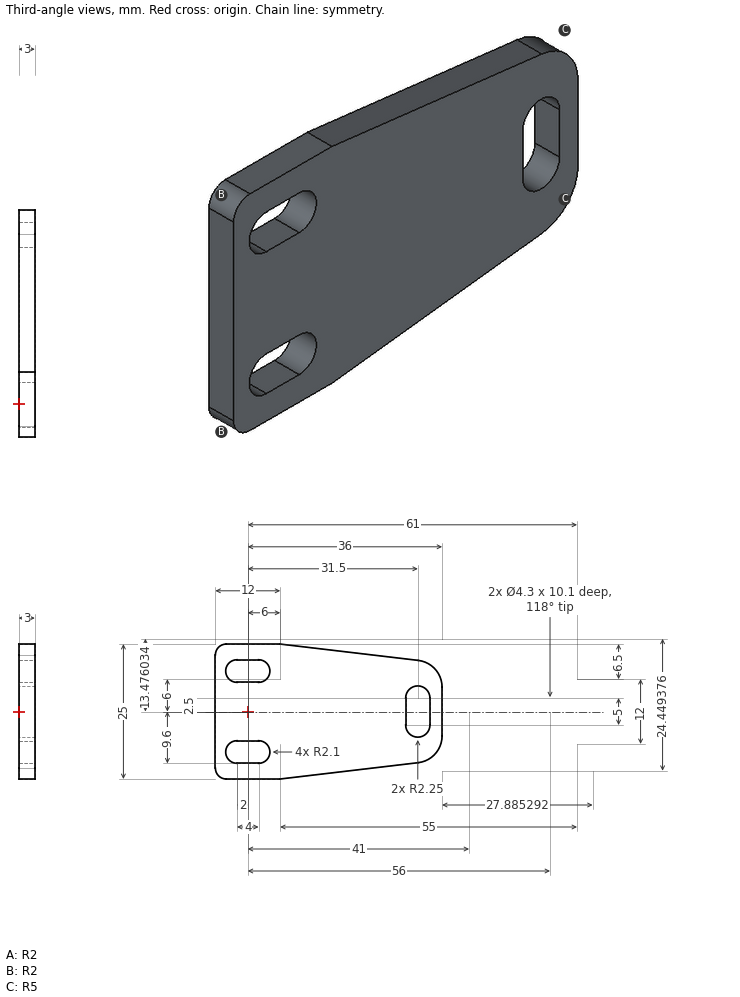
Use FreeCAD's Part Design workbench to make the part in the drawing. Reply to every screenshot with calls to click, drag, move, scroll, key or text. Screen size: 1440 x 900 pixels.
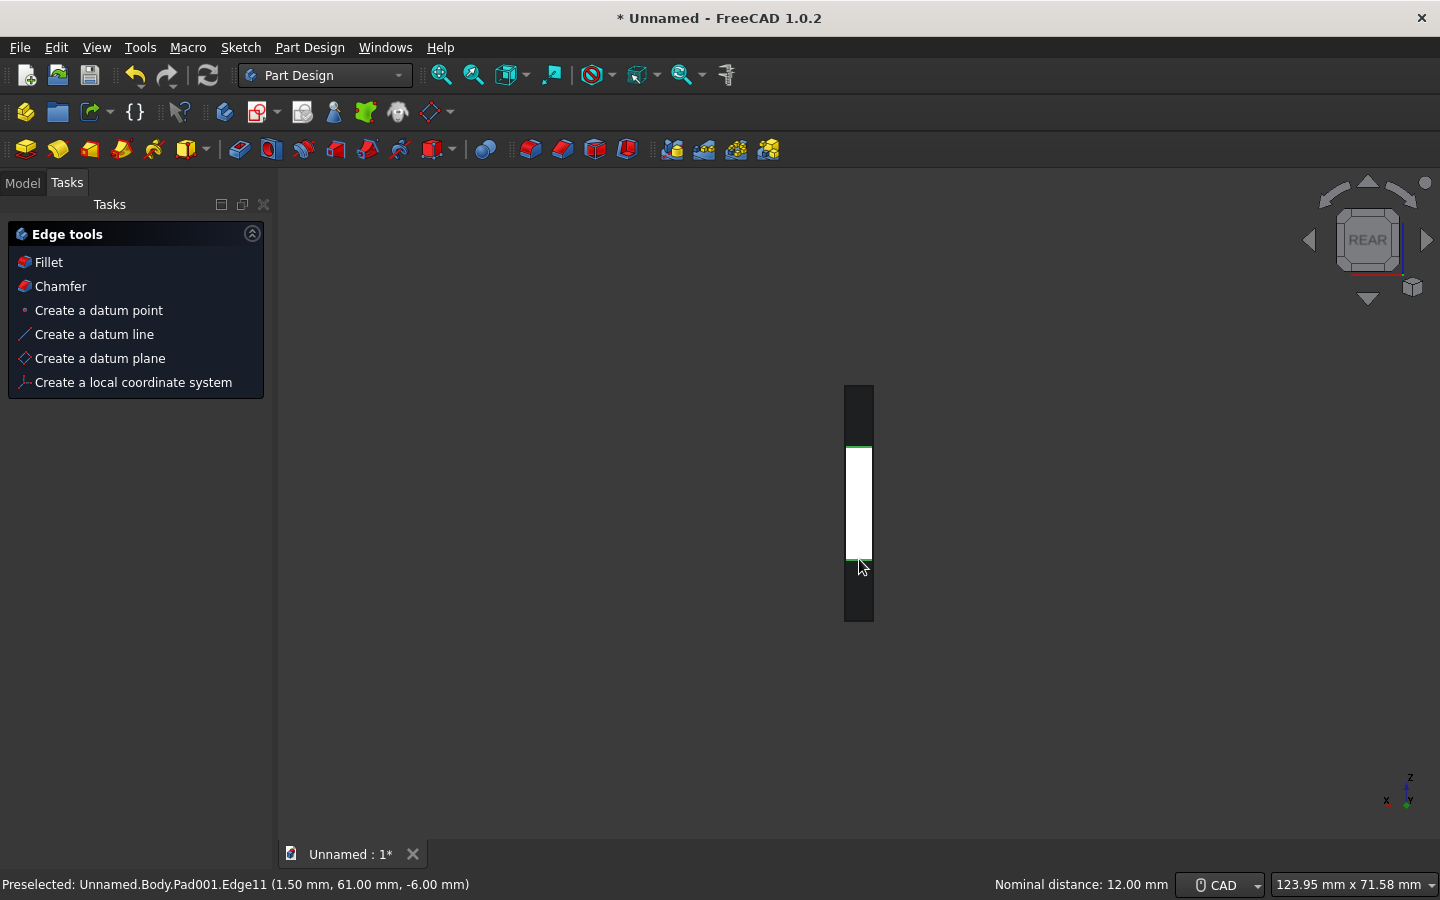
click(532, 150)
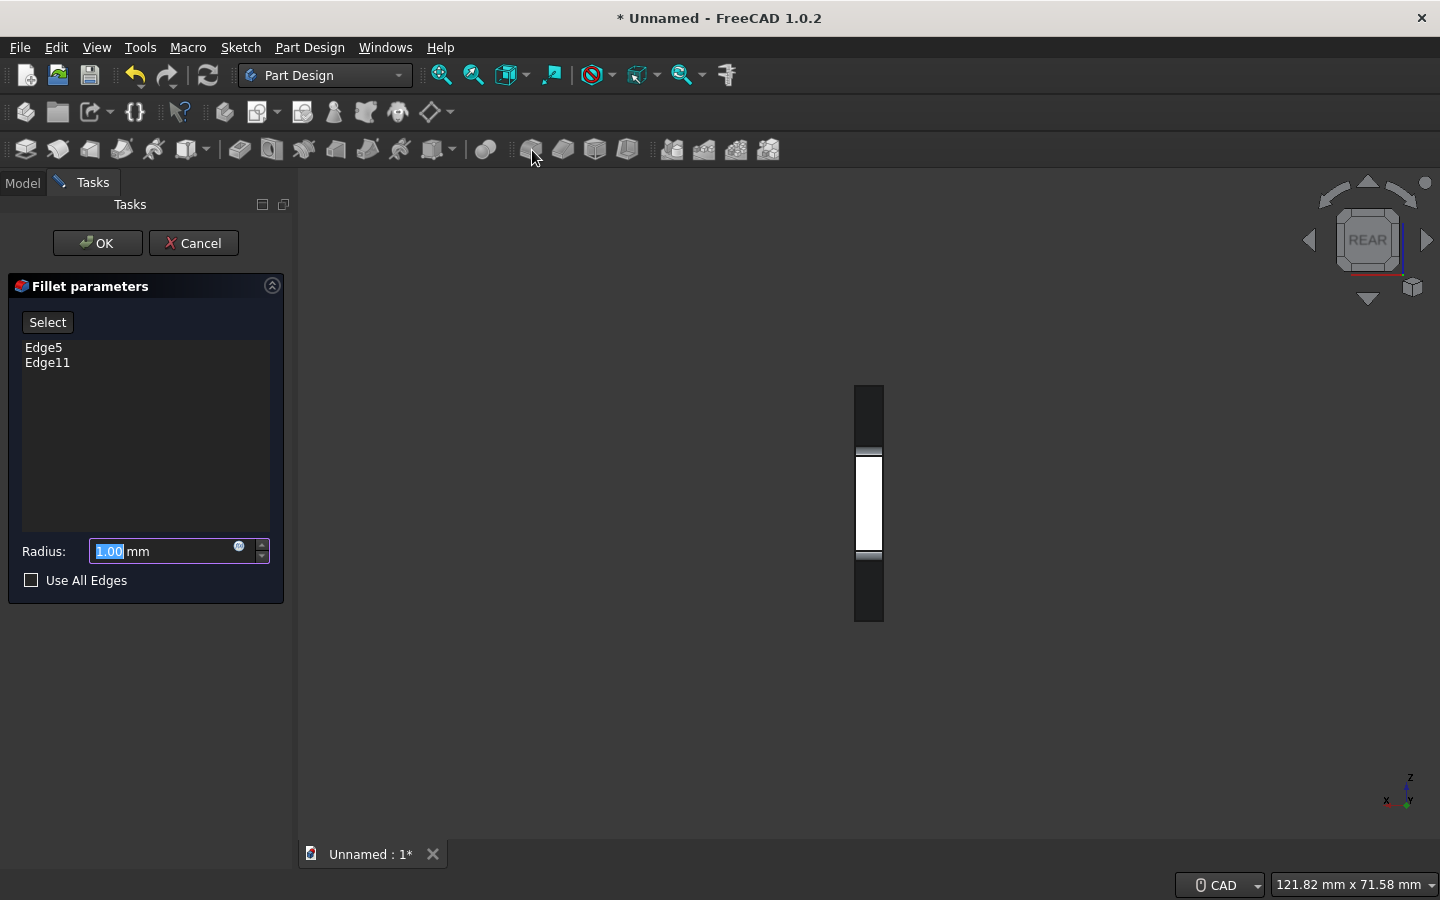
text(2)
key(Tab)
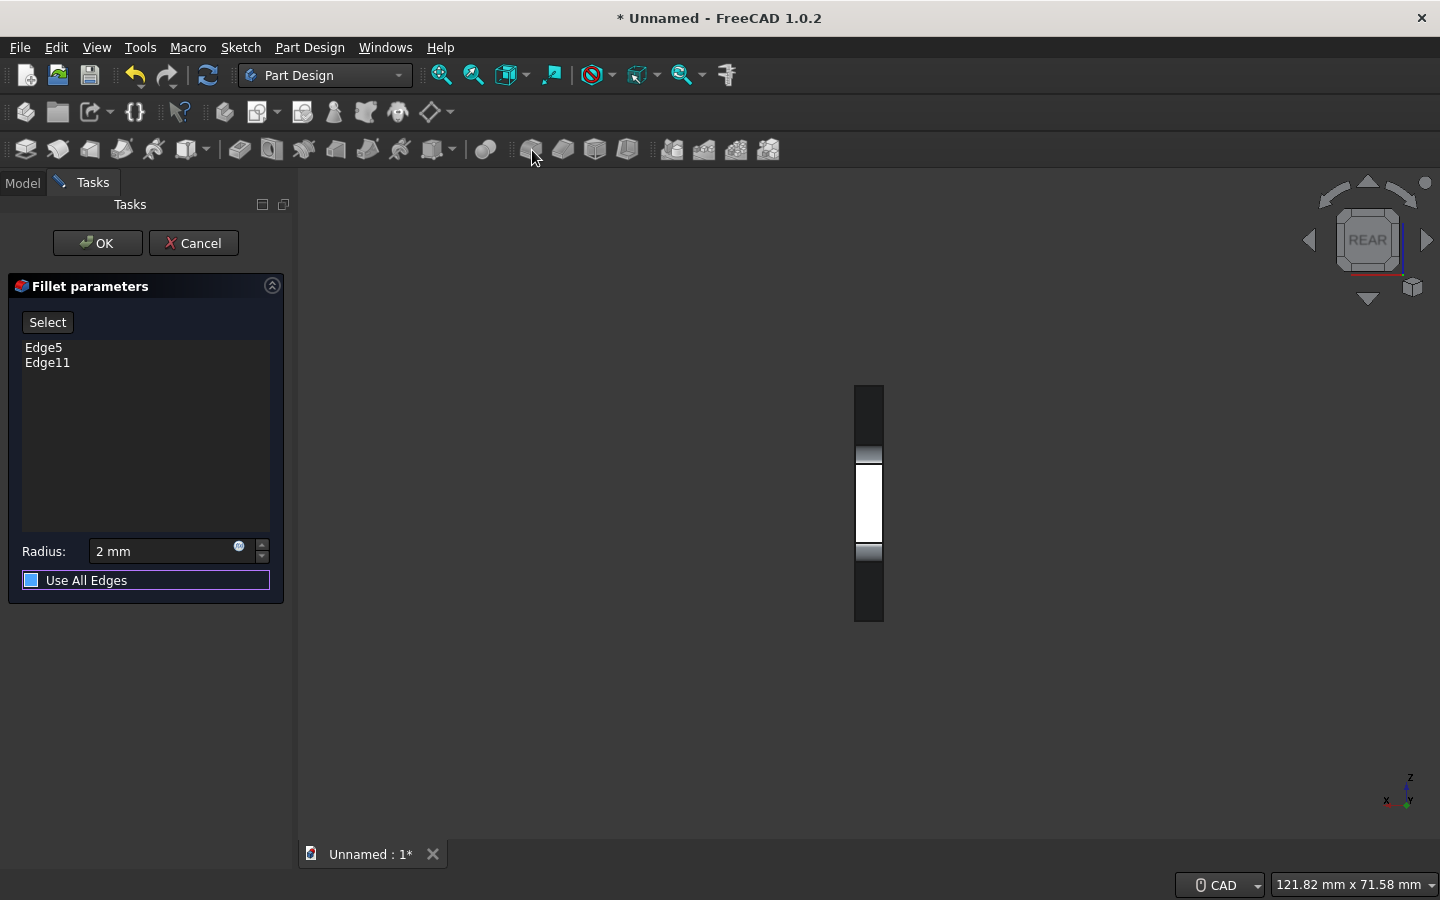
click(98, 243)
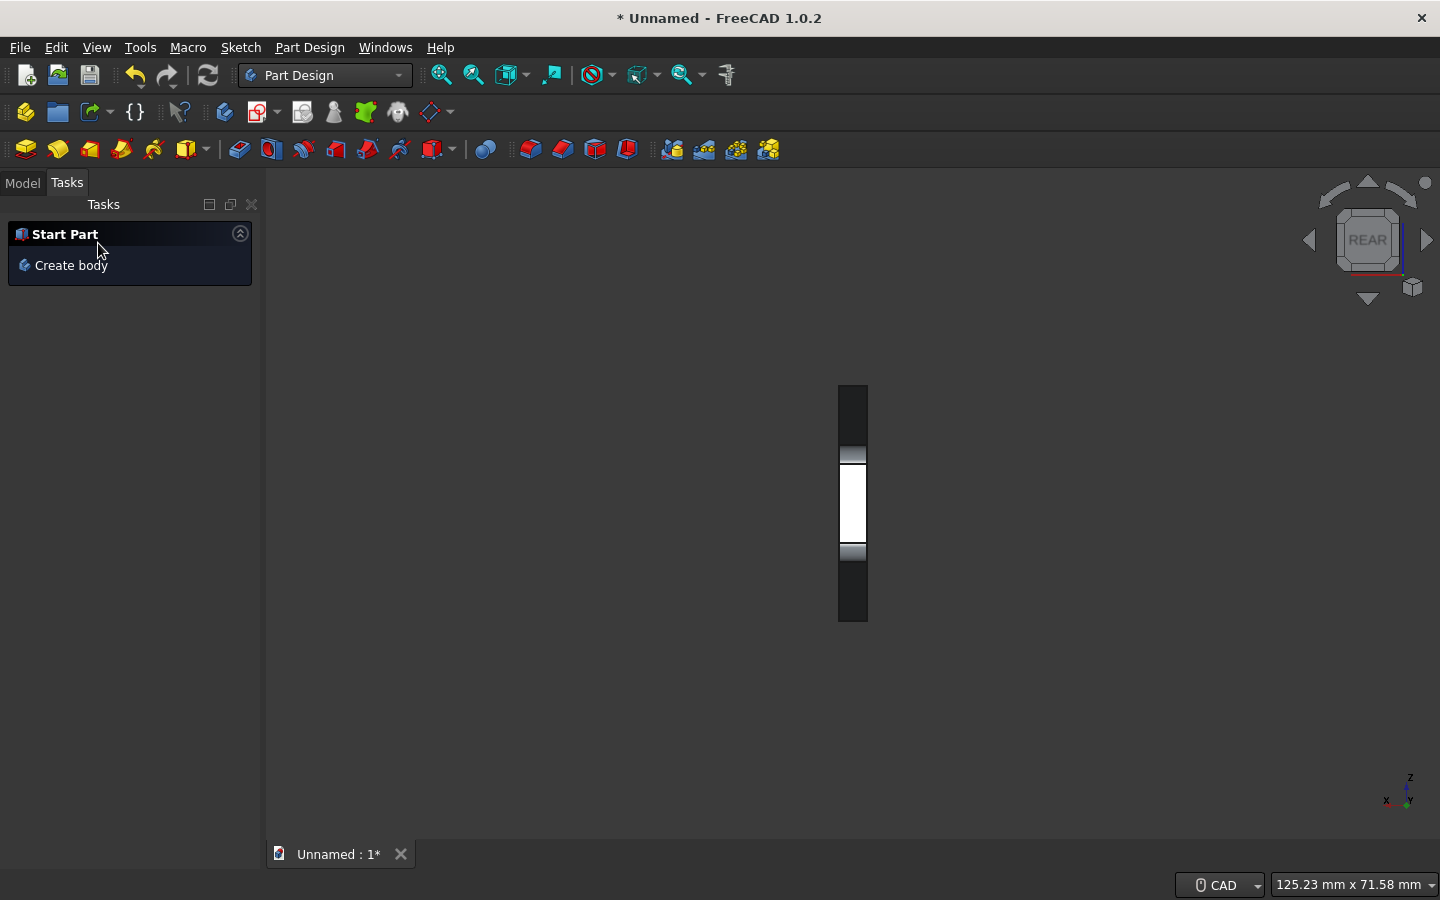
key(v)
key(f)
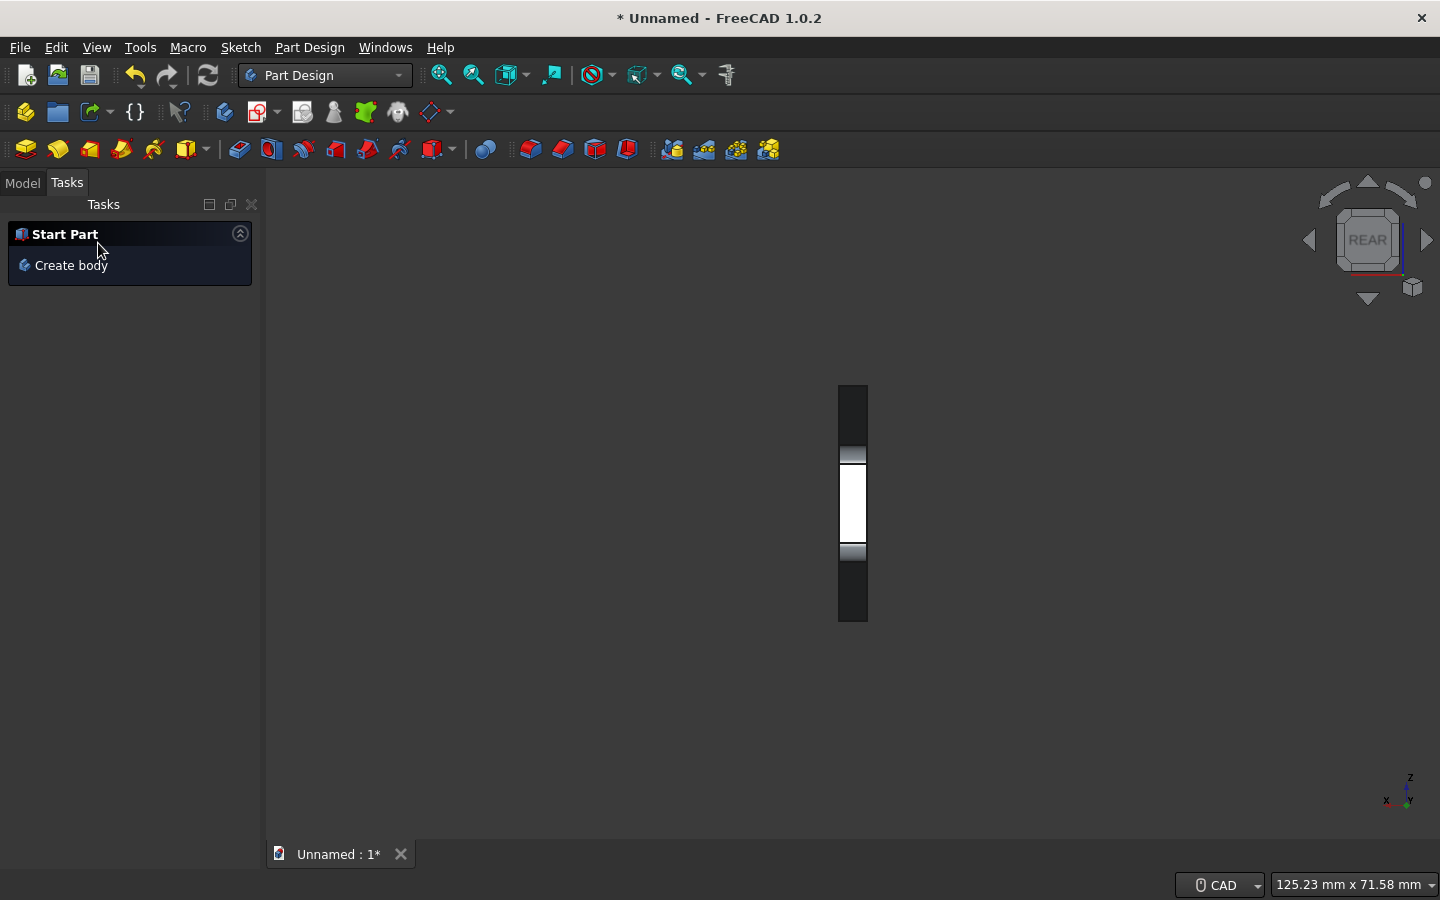
key(6)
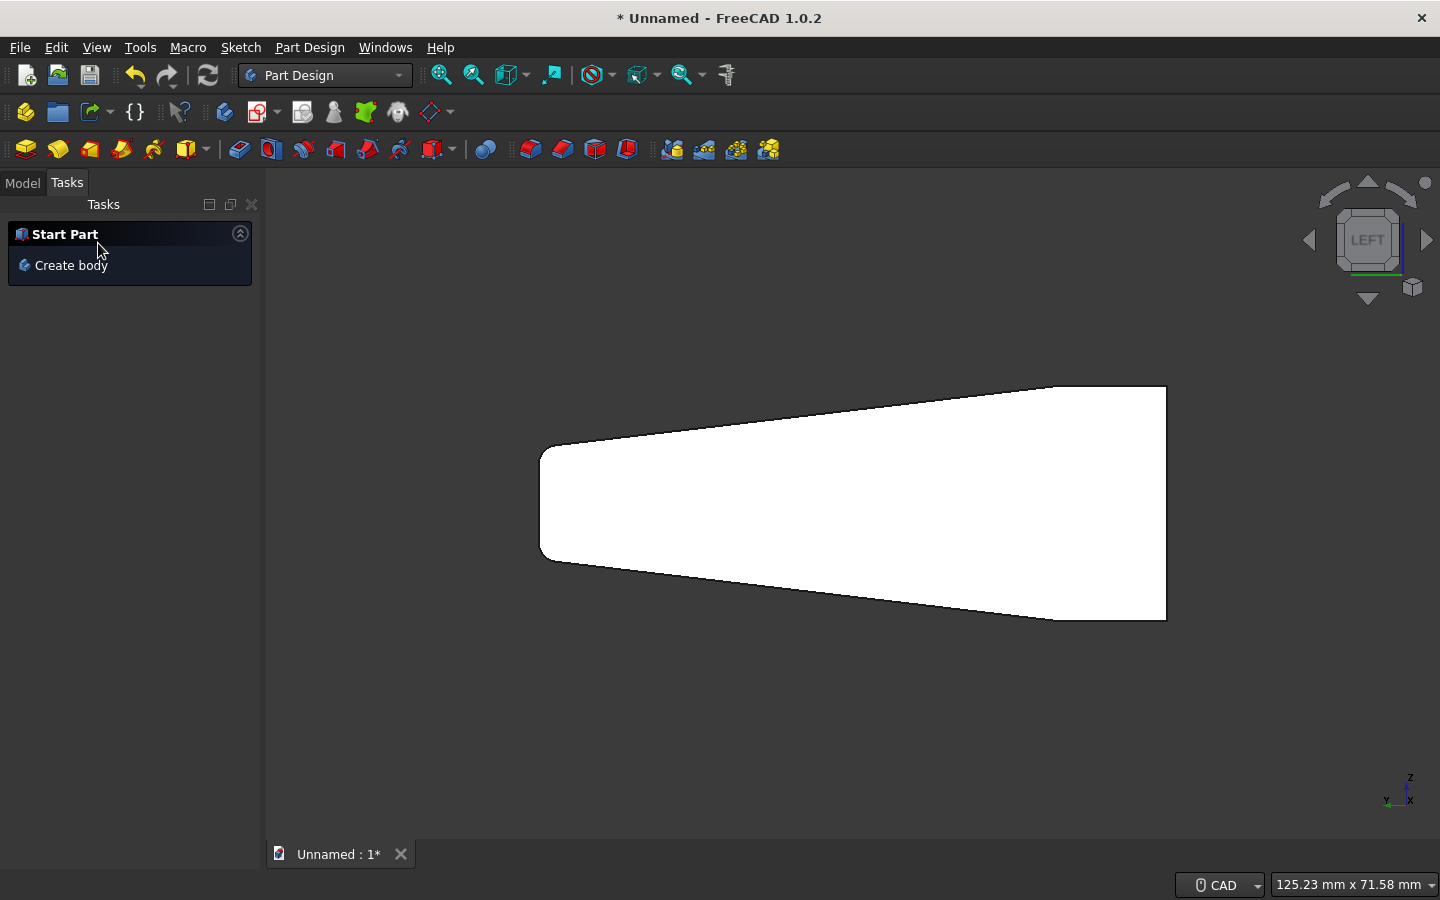
click(1032, 502)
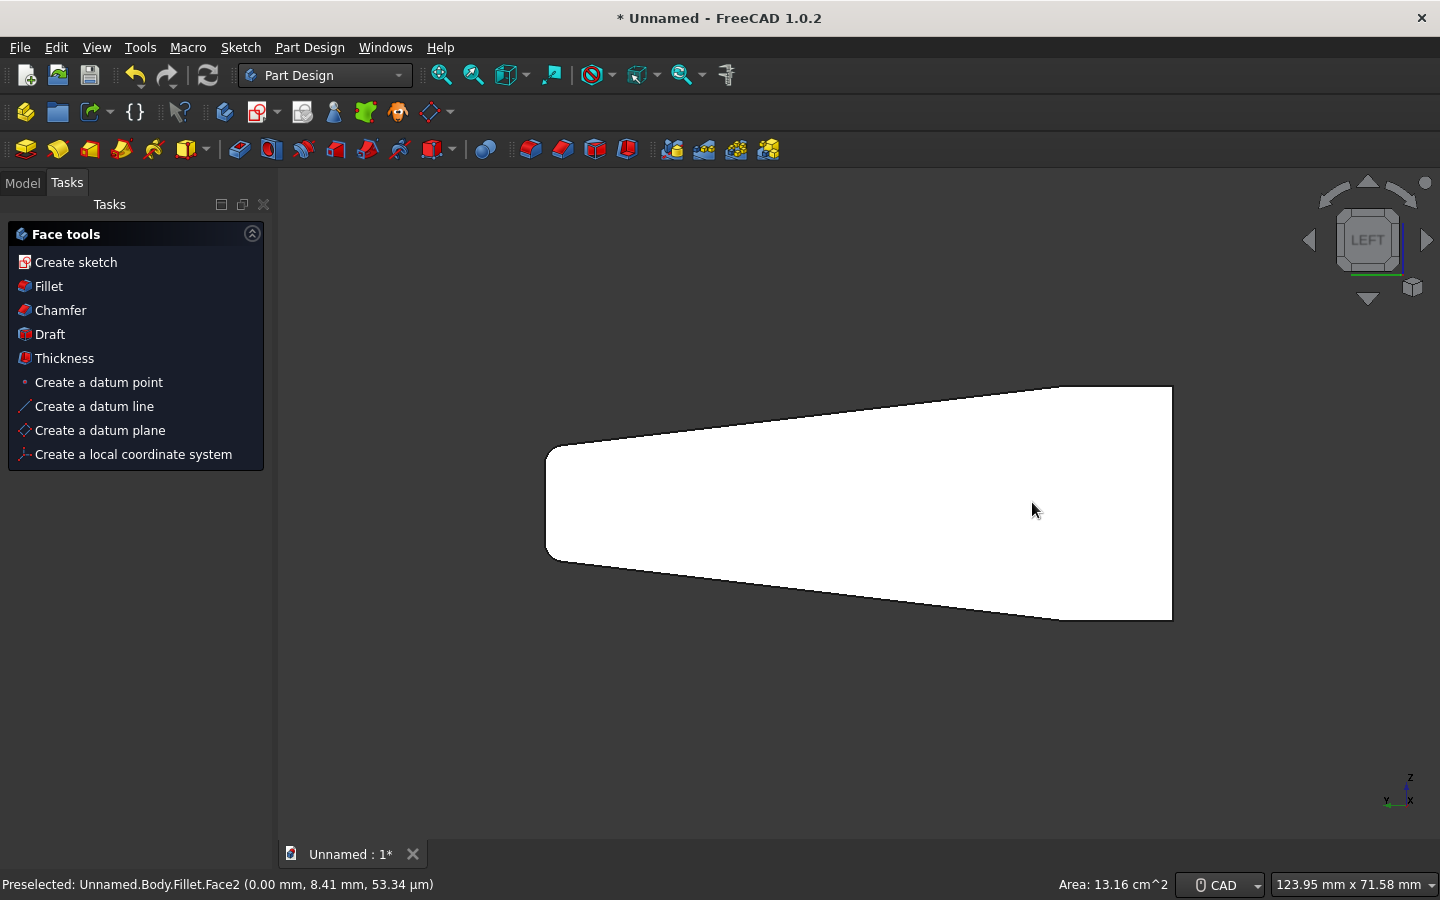
click(258, 112)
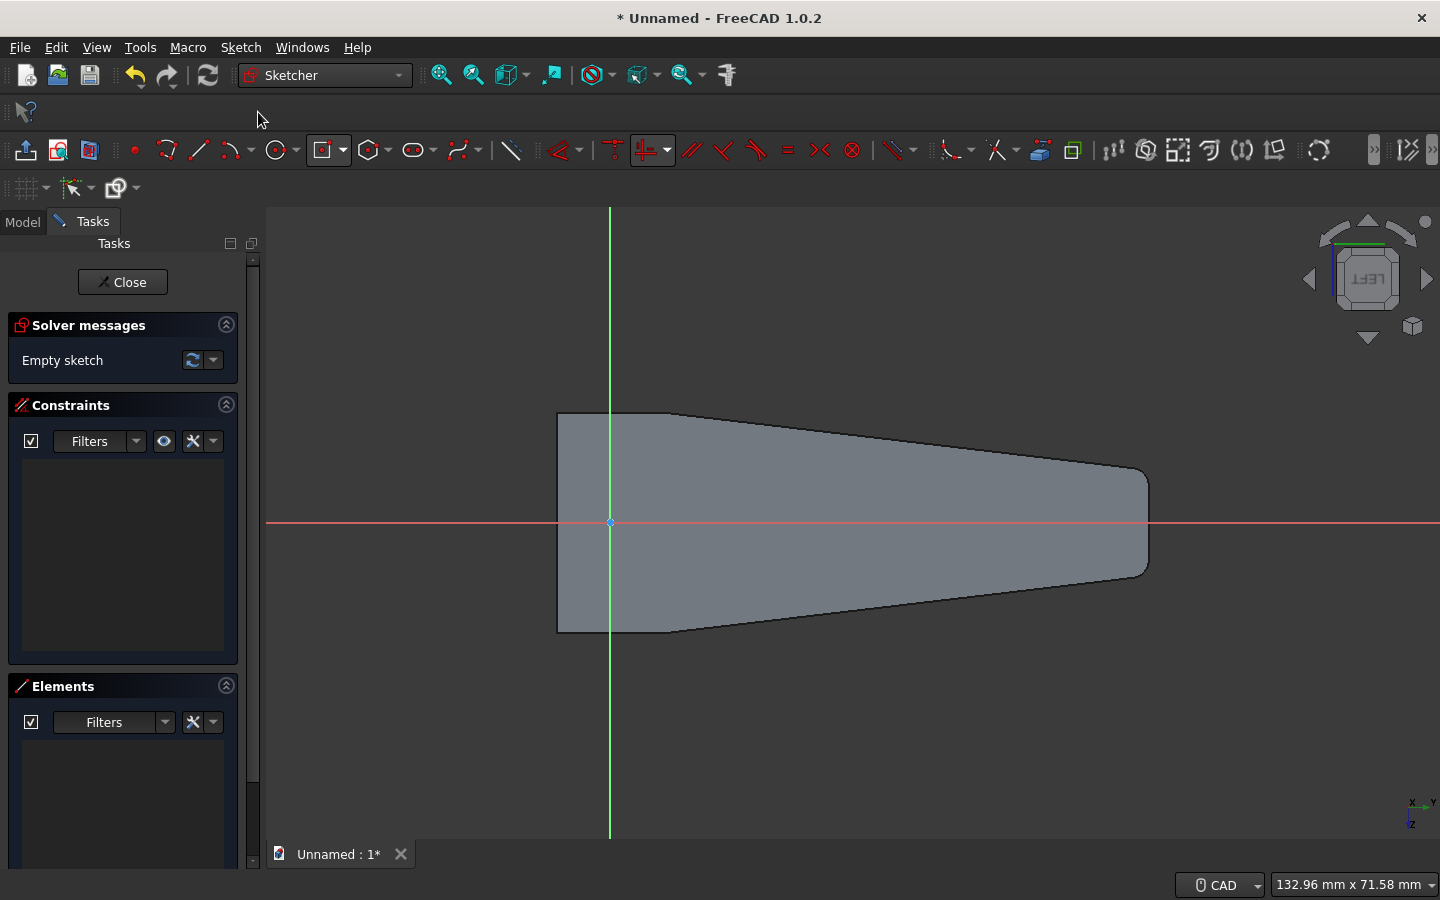
scroll(468, 523, up, 4)